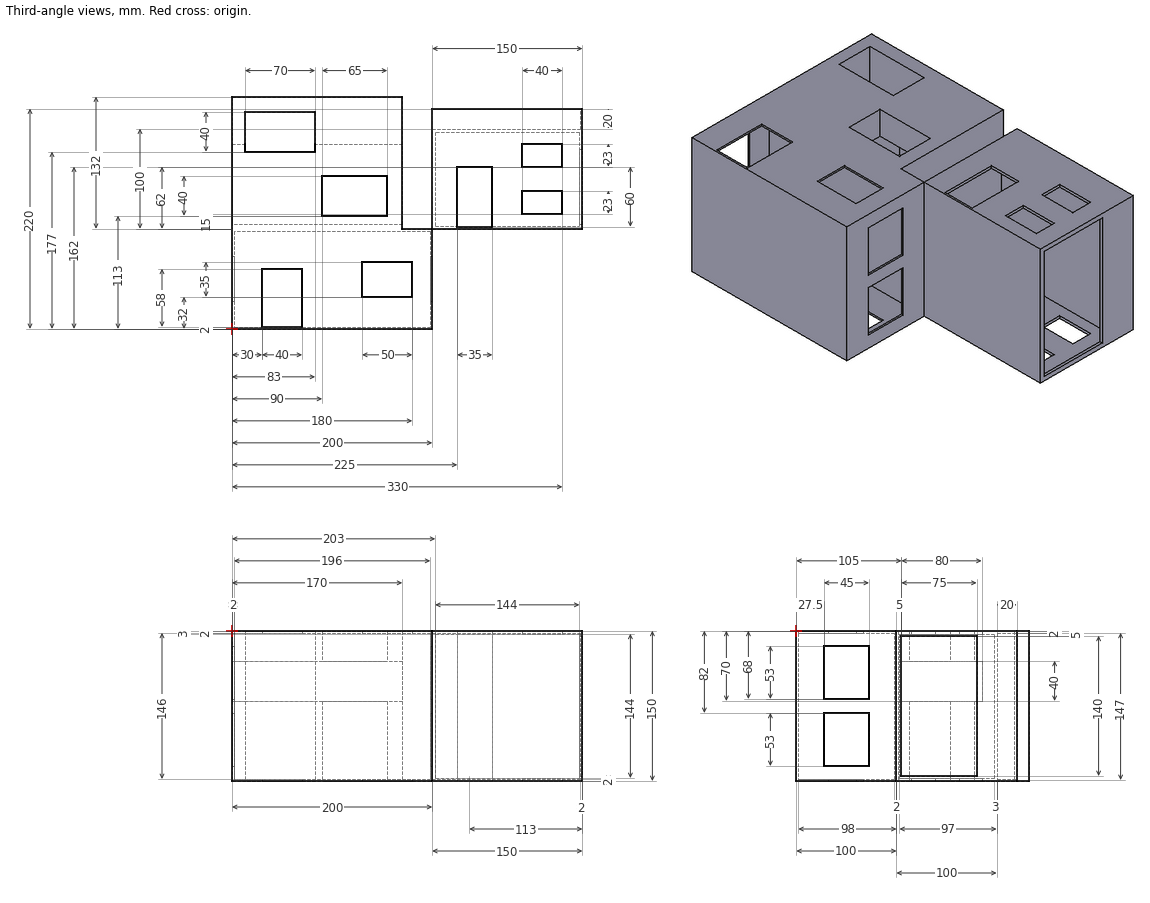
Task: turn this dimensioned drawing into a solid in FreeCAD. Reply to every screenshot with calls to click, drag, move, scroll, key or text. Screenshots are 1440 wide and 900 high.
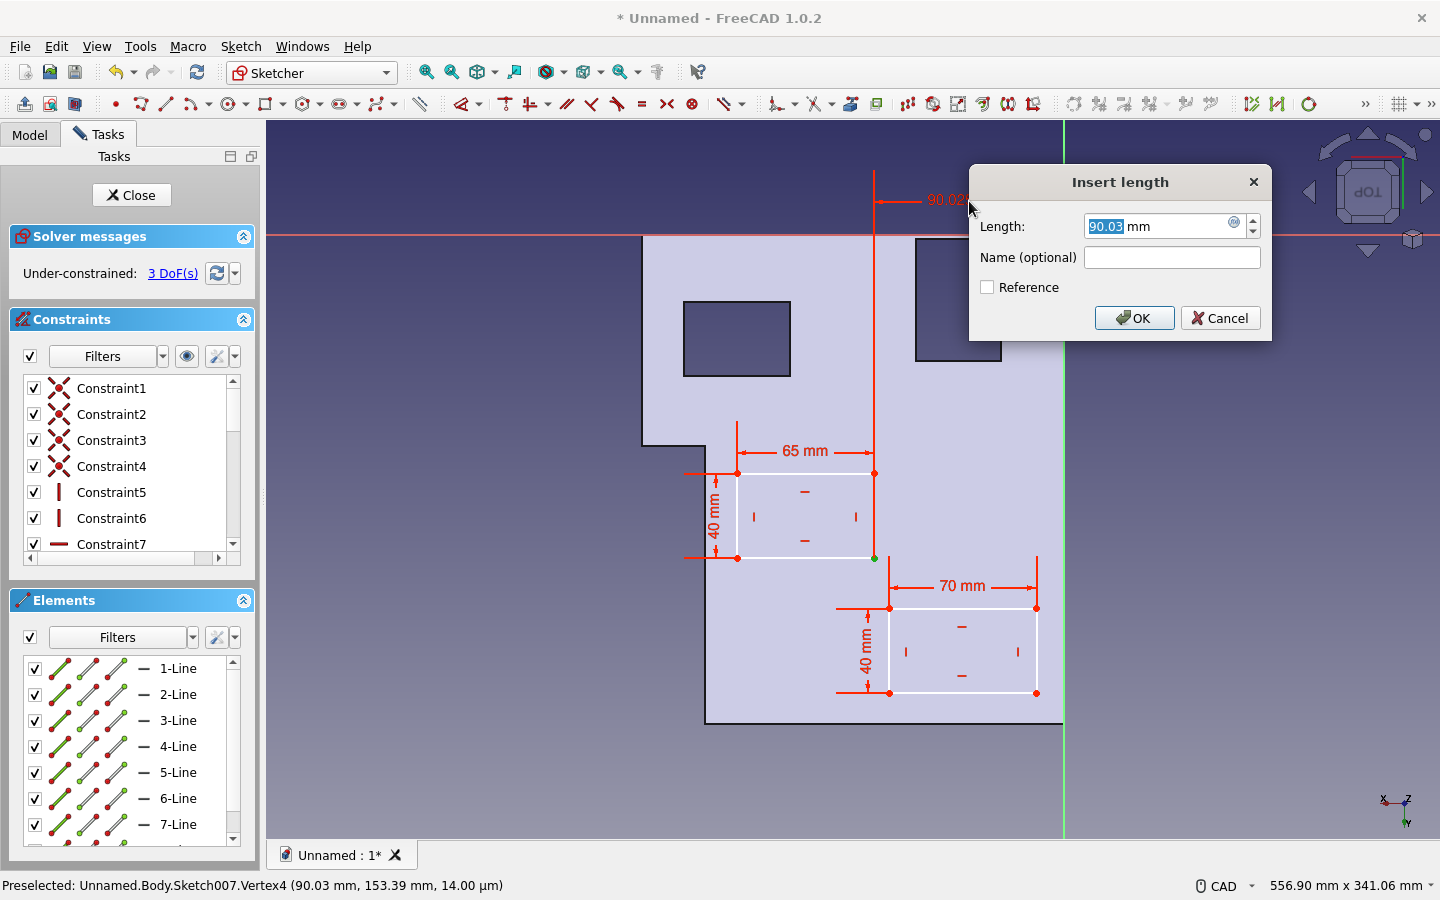
text(90)
key(Return)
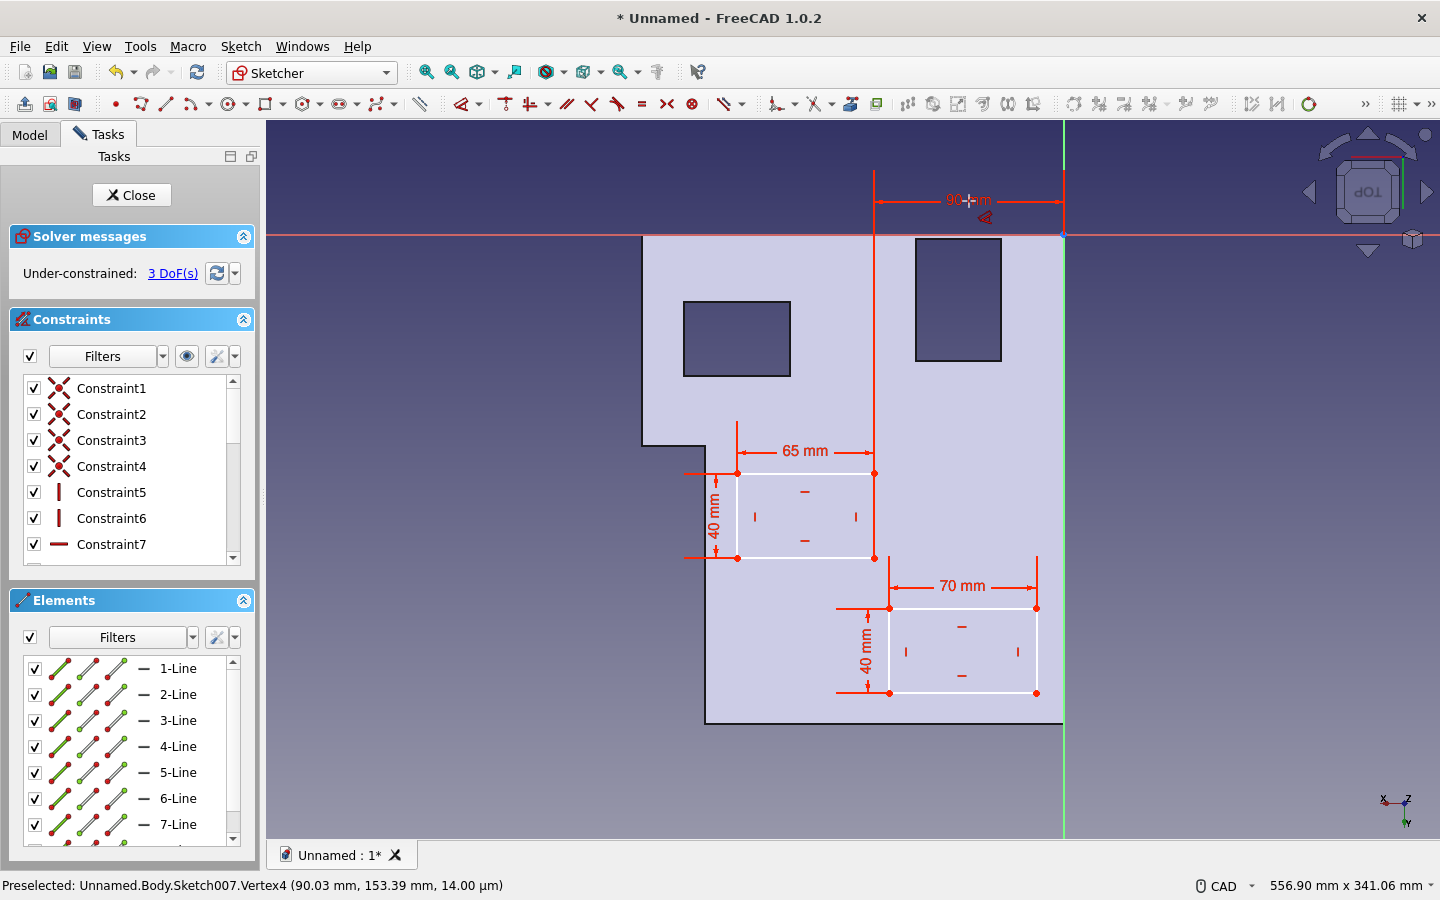
click(889, 609)
click(976, 643)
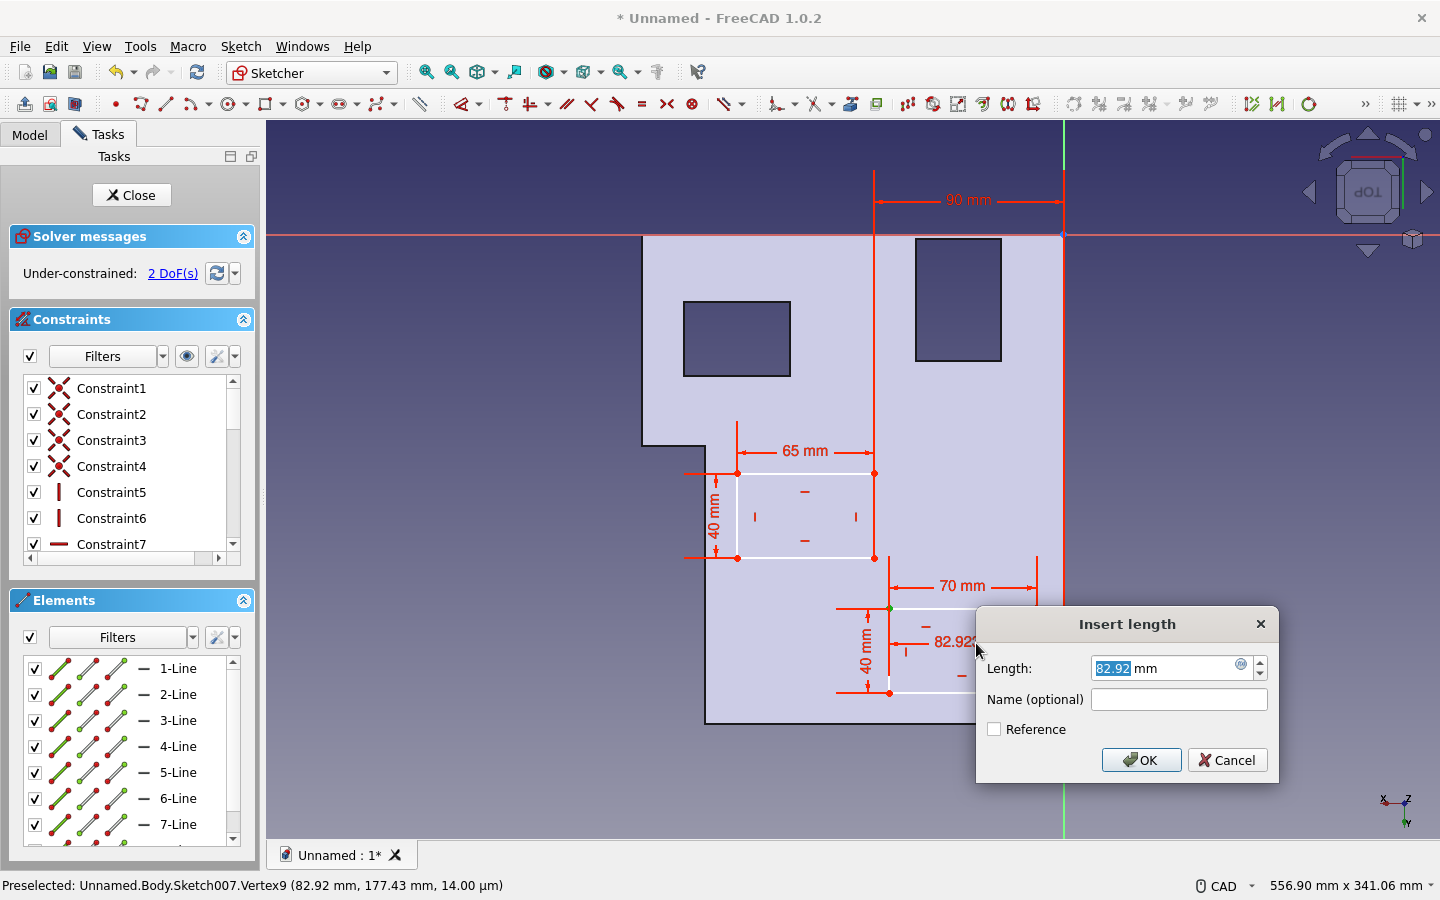
text(83)
key(Return)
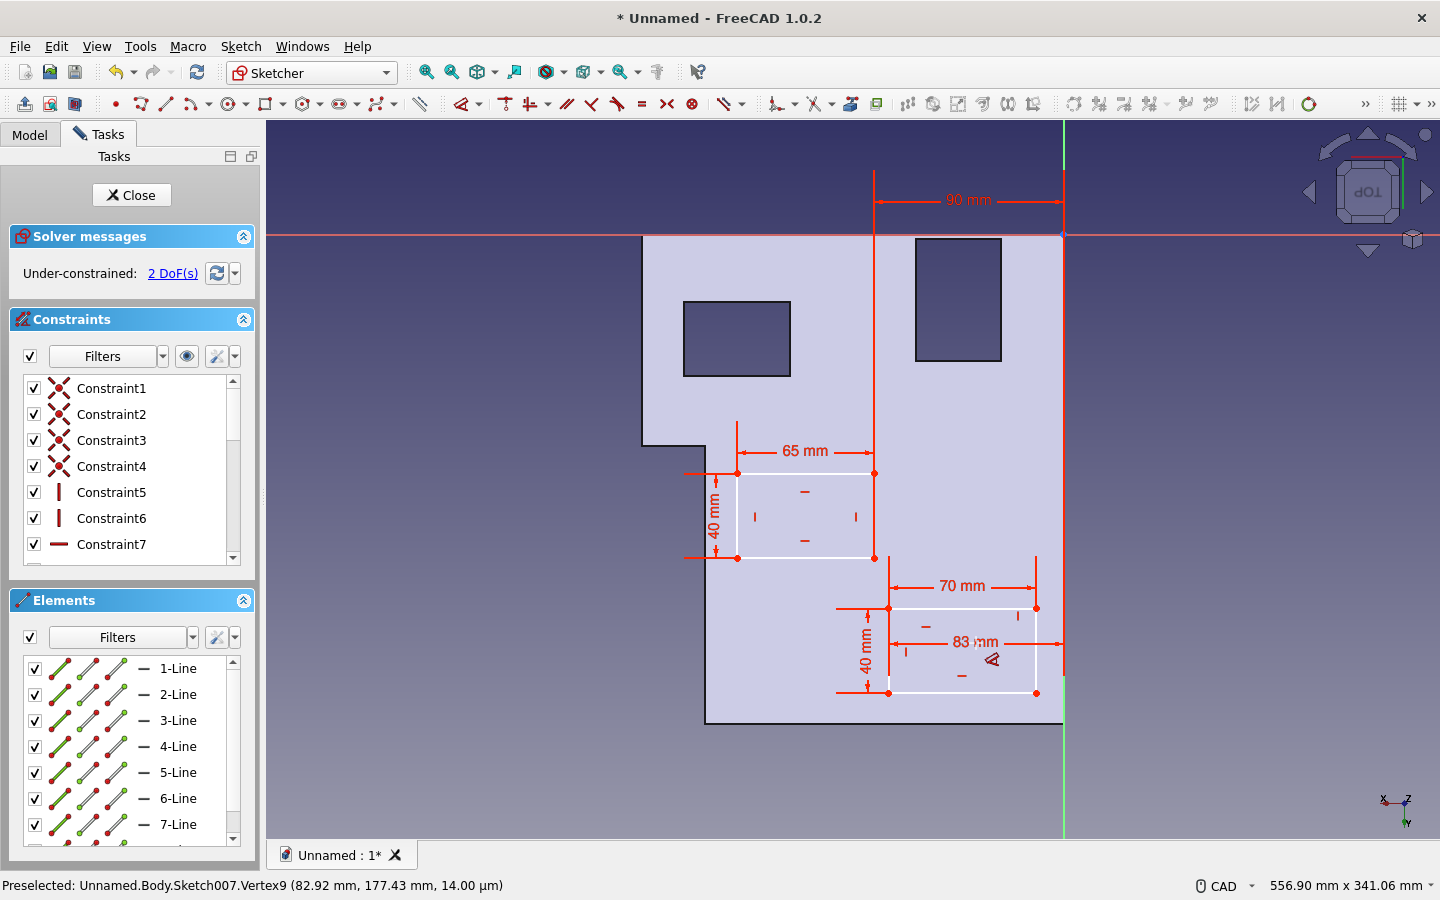
click(737, 474)
click(1098, 354)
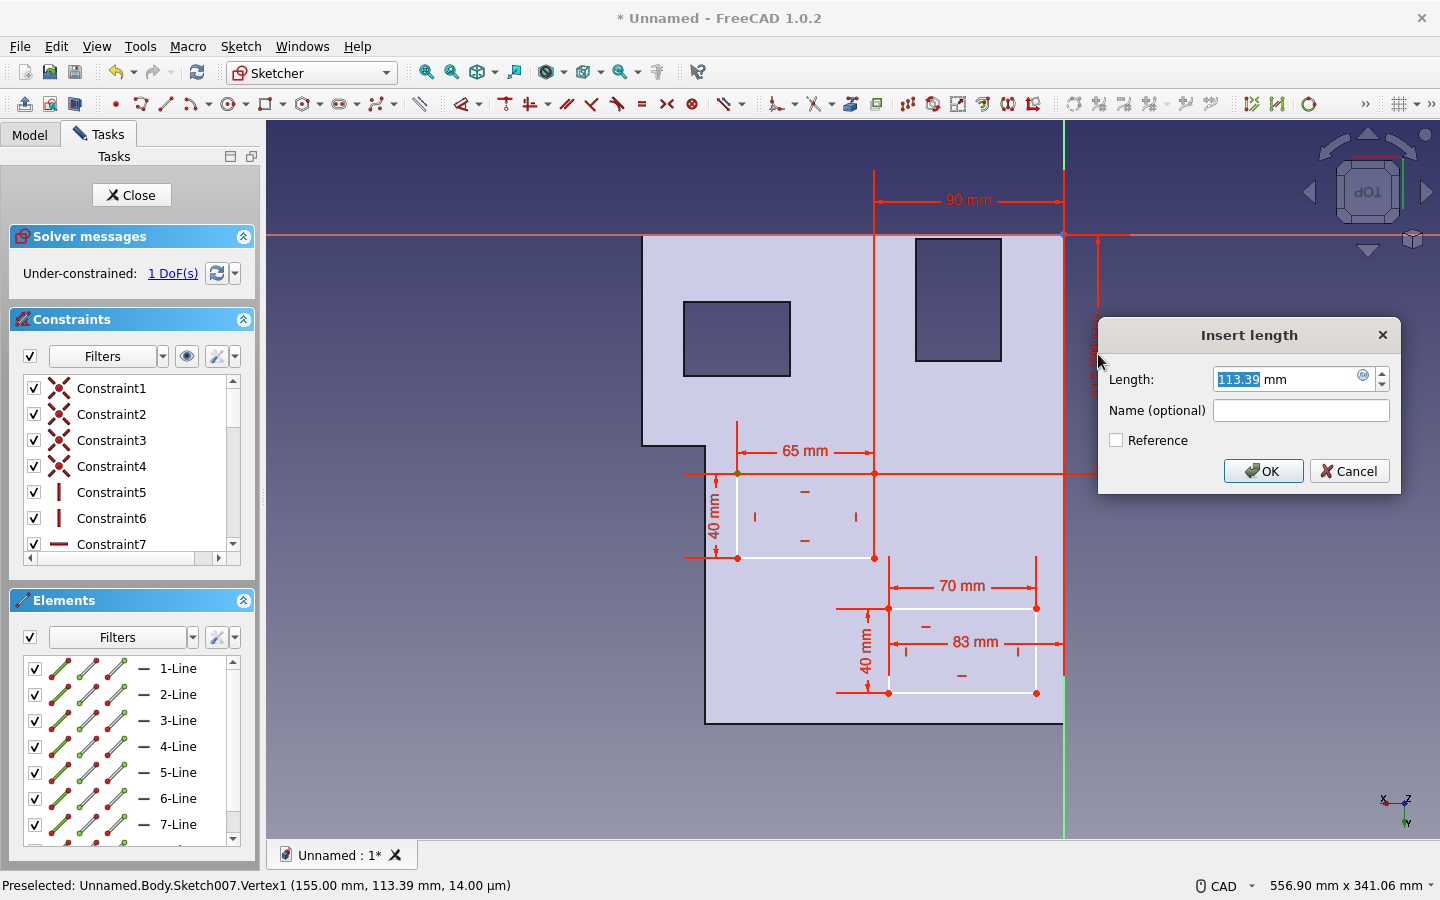
text(113)
key(Return)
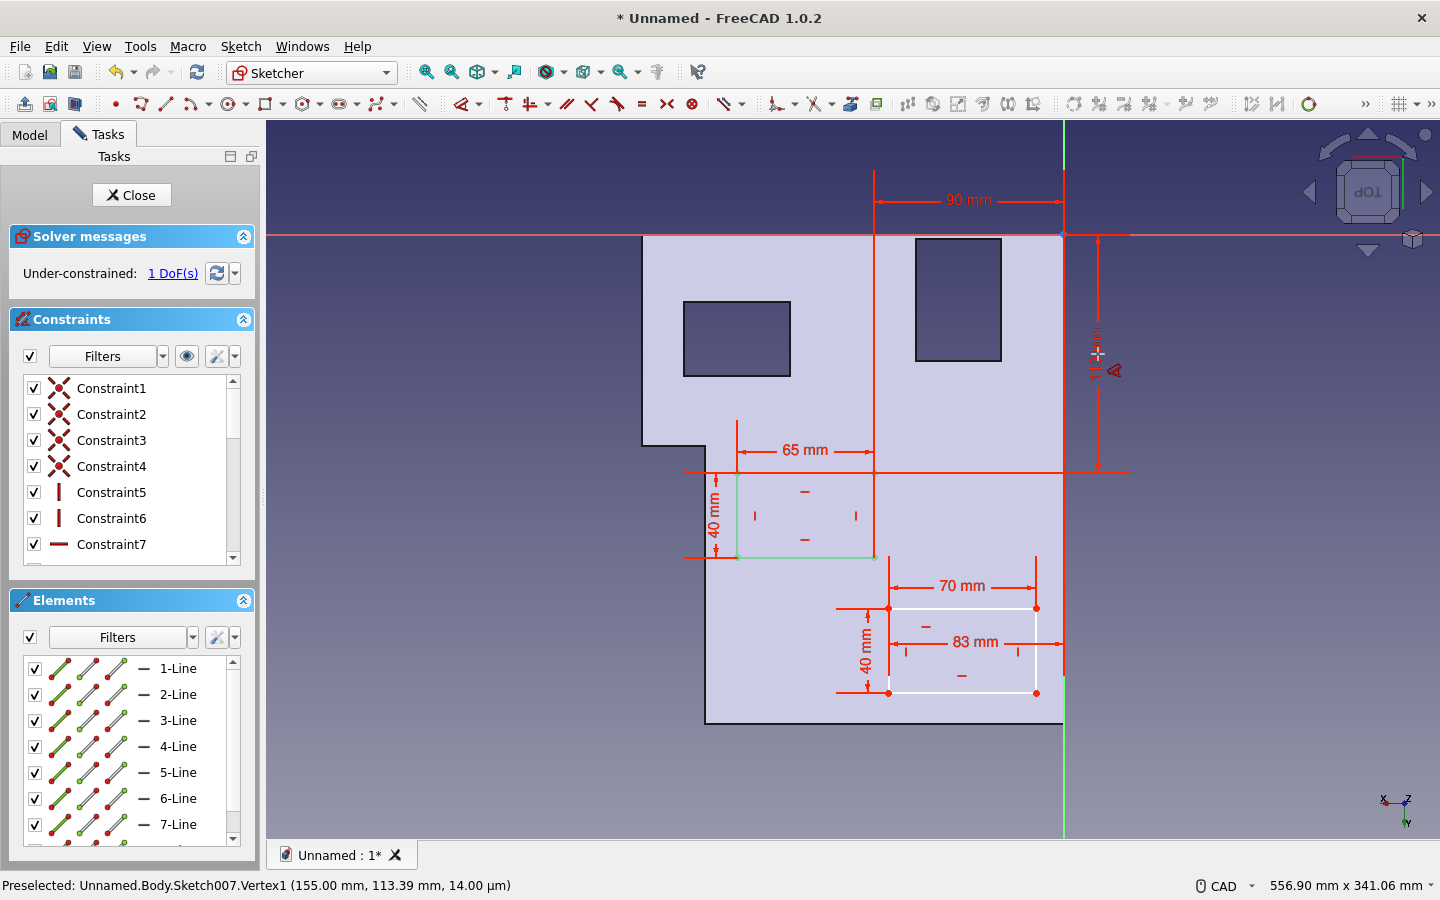
click(889, 609)
click(1098, 422)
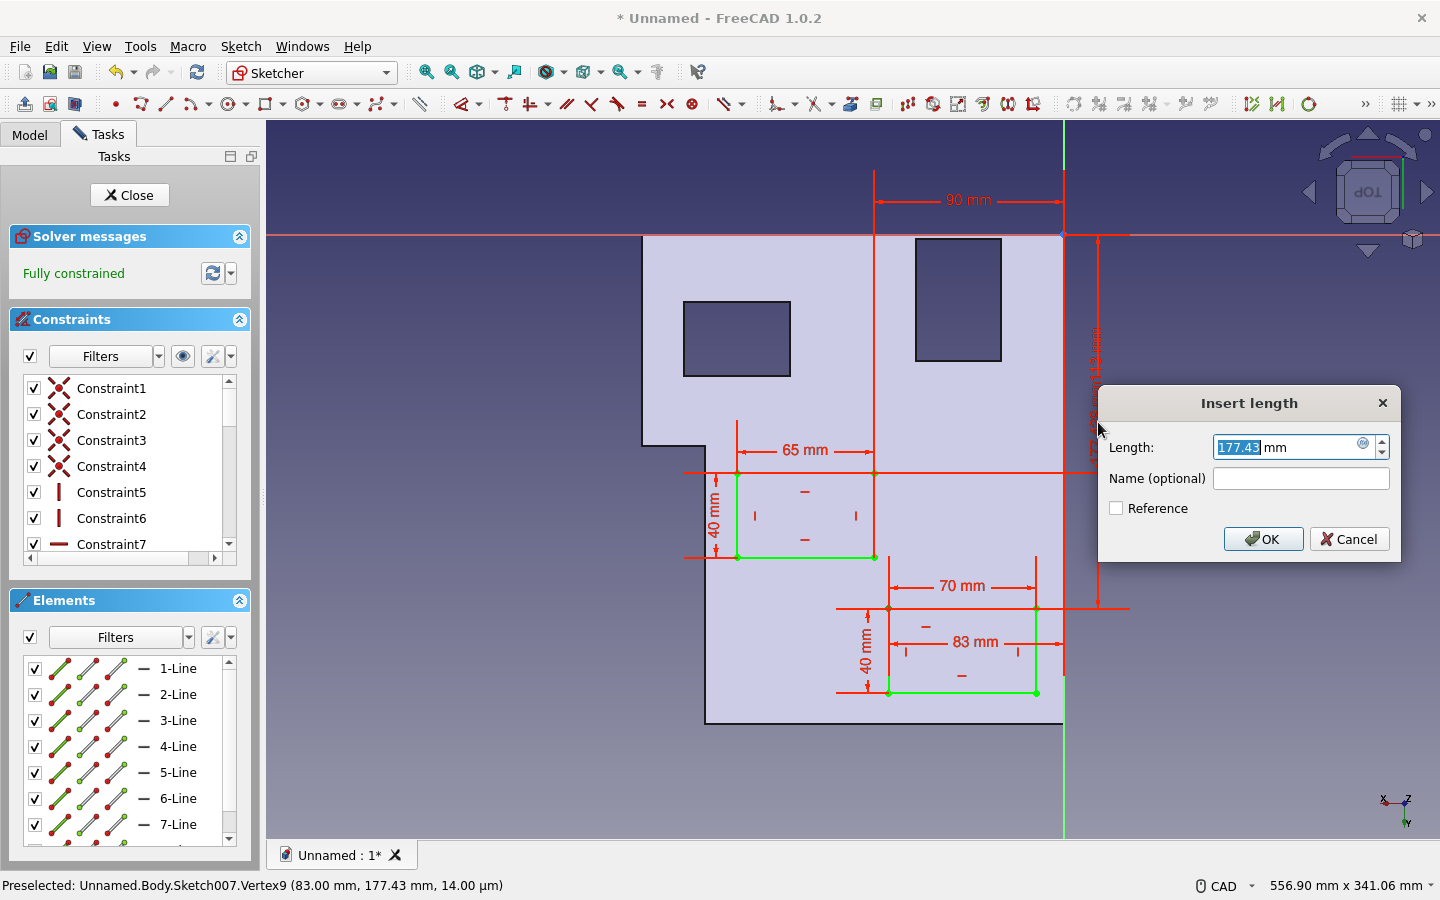
text(177)
key(Return)
key(Escape)